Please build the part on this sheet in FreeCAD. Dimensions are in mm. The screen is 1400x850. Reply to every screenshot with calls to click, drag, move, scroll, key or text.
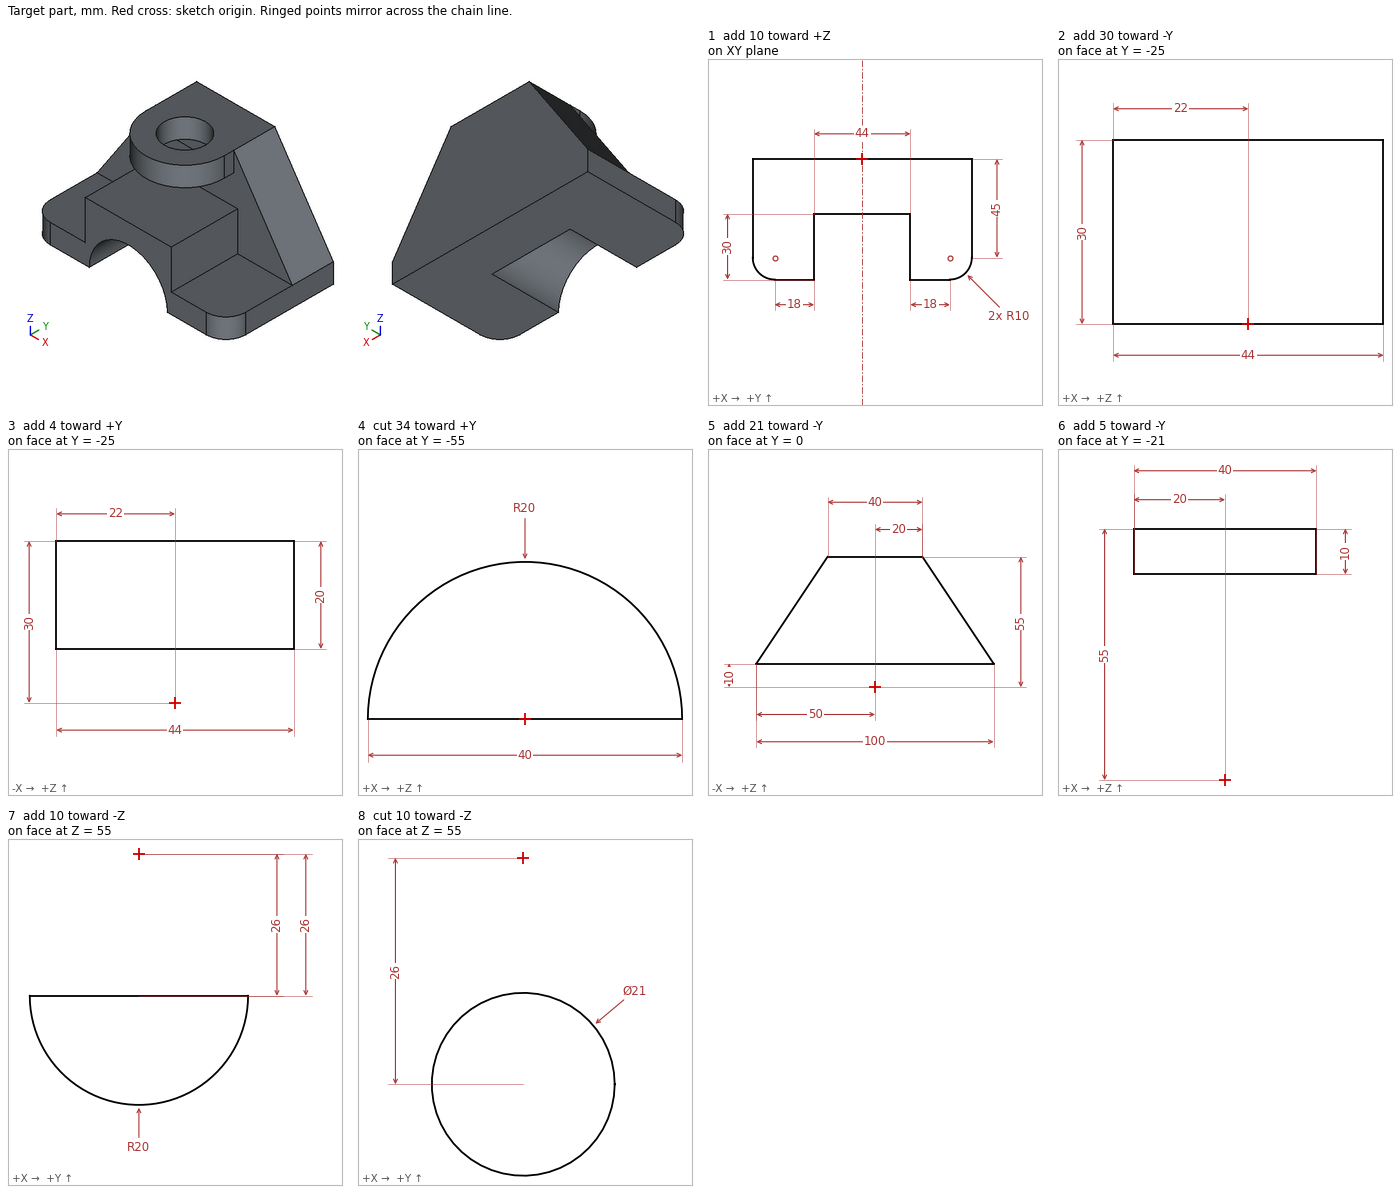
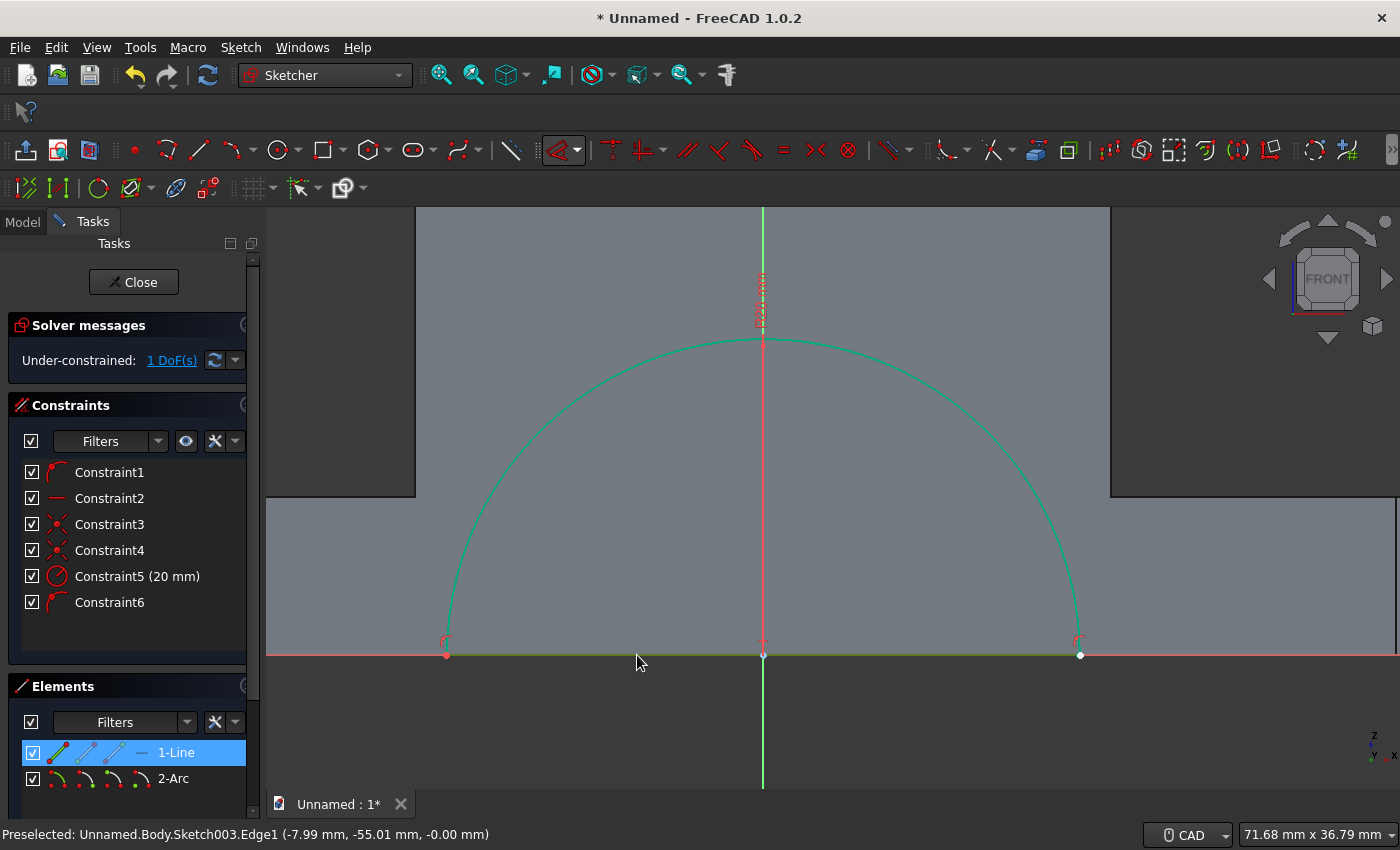
click(580, 150)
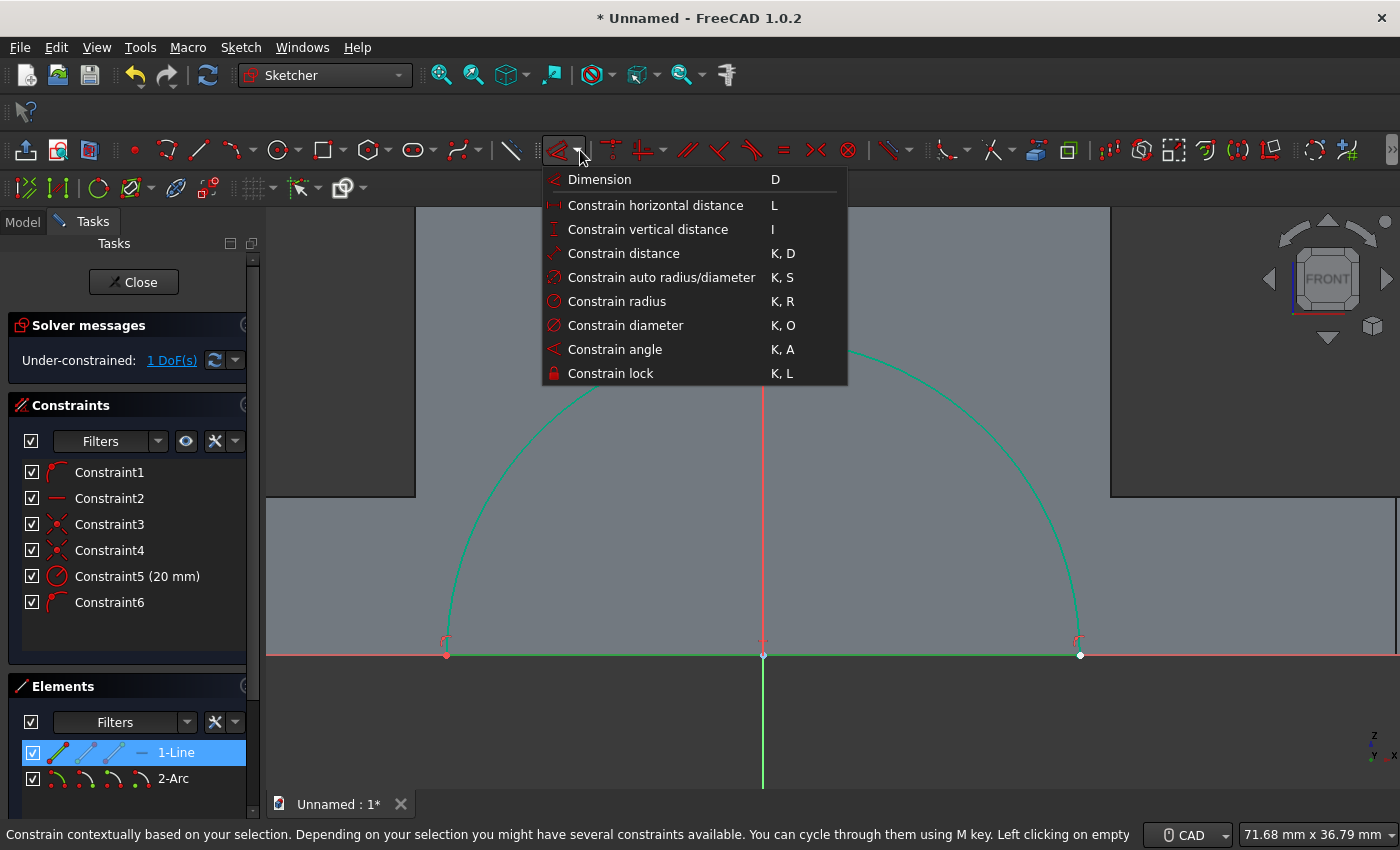
click(695, 205)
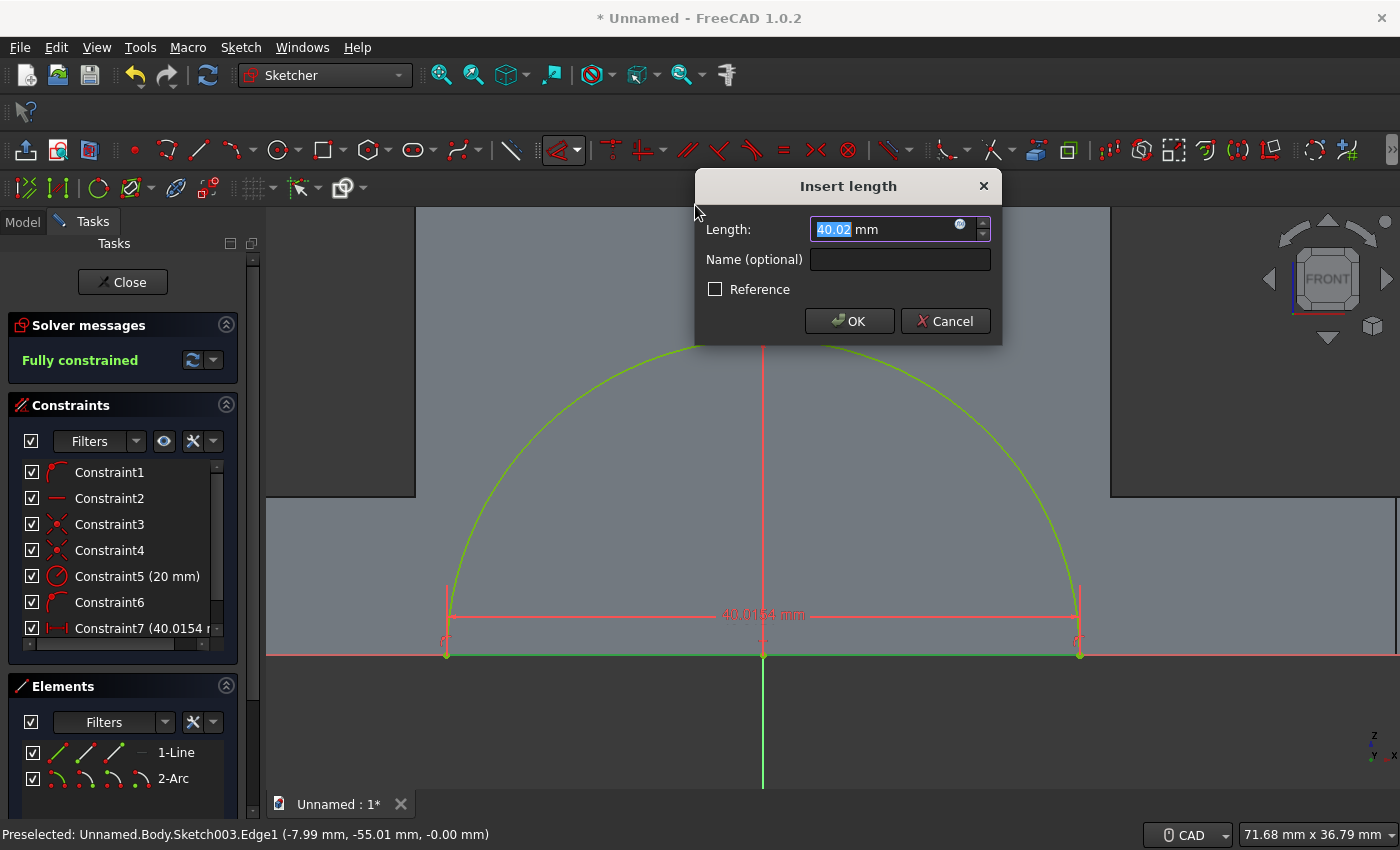
text(40)
key(Return)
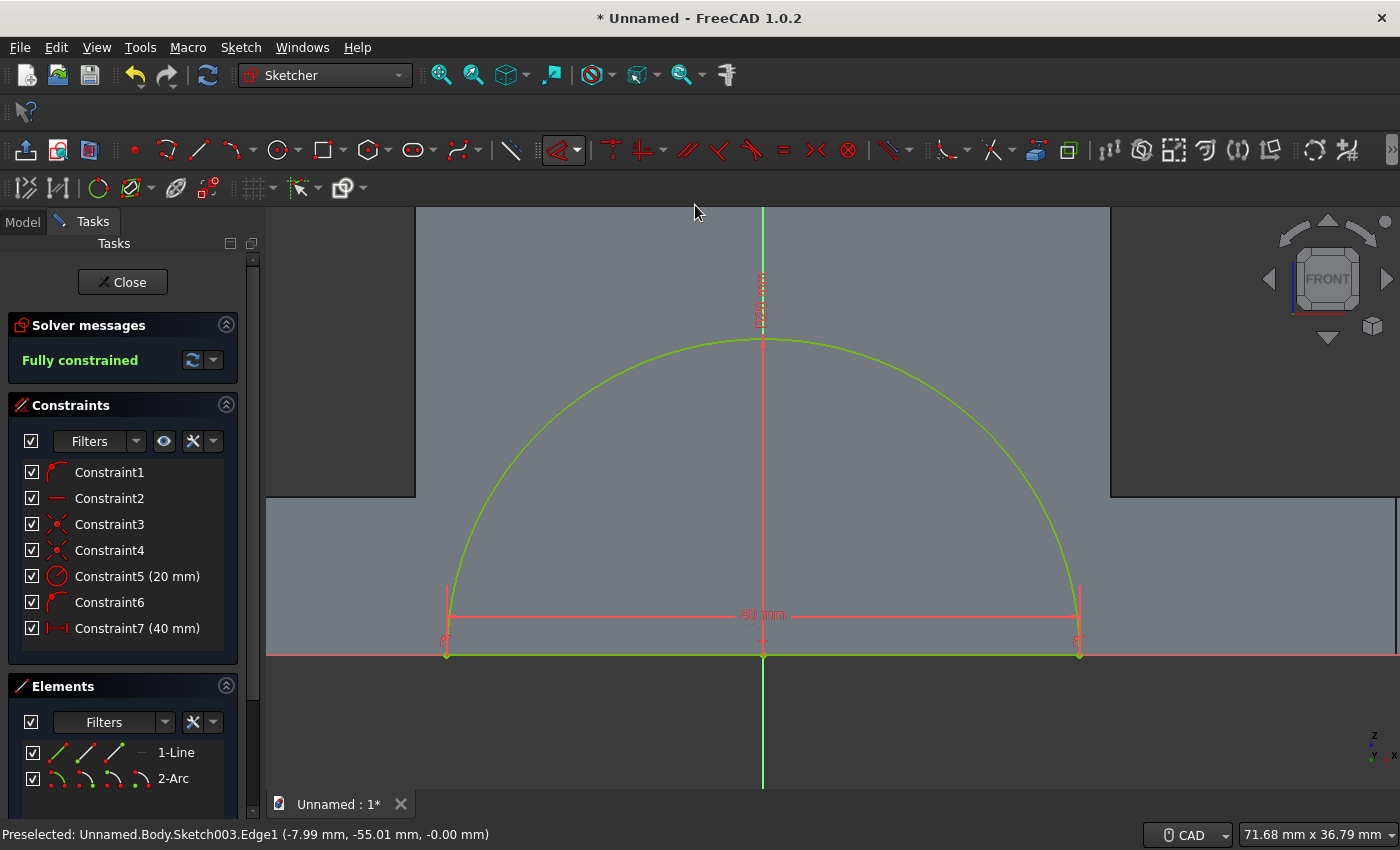
click(123, 282)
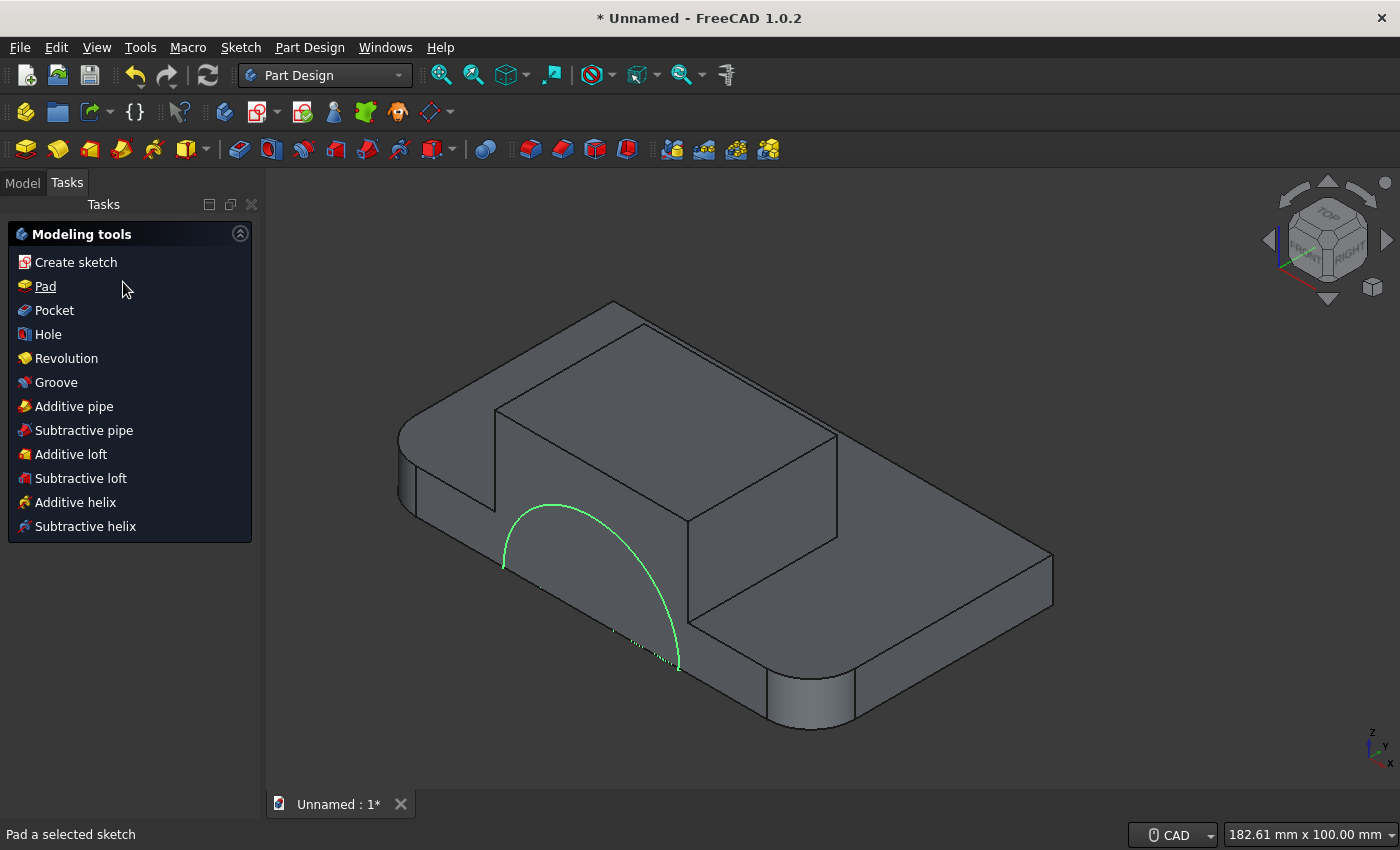
click(240, 150)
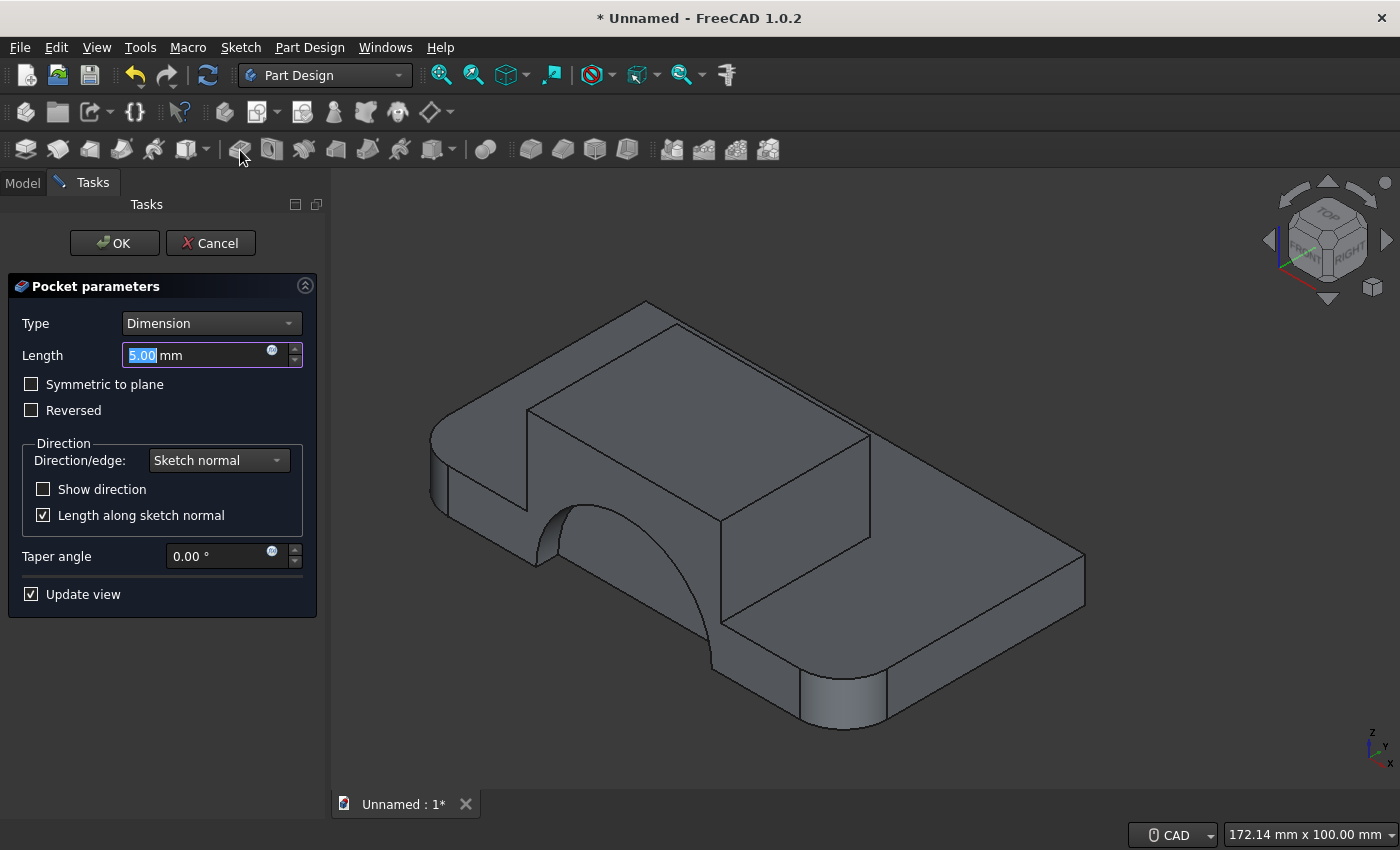
text(34)
key(Tab)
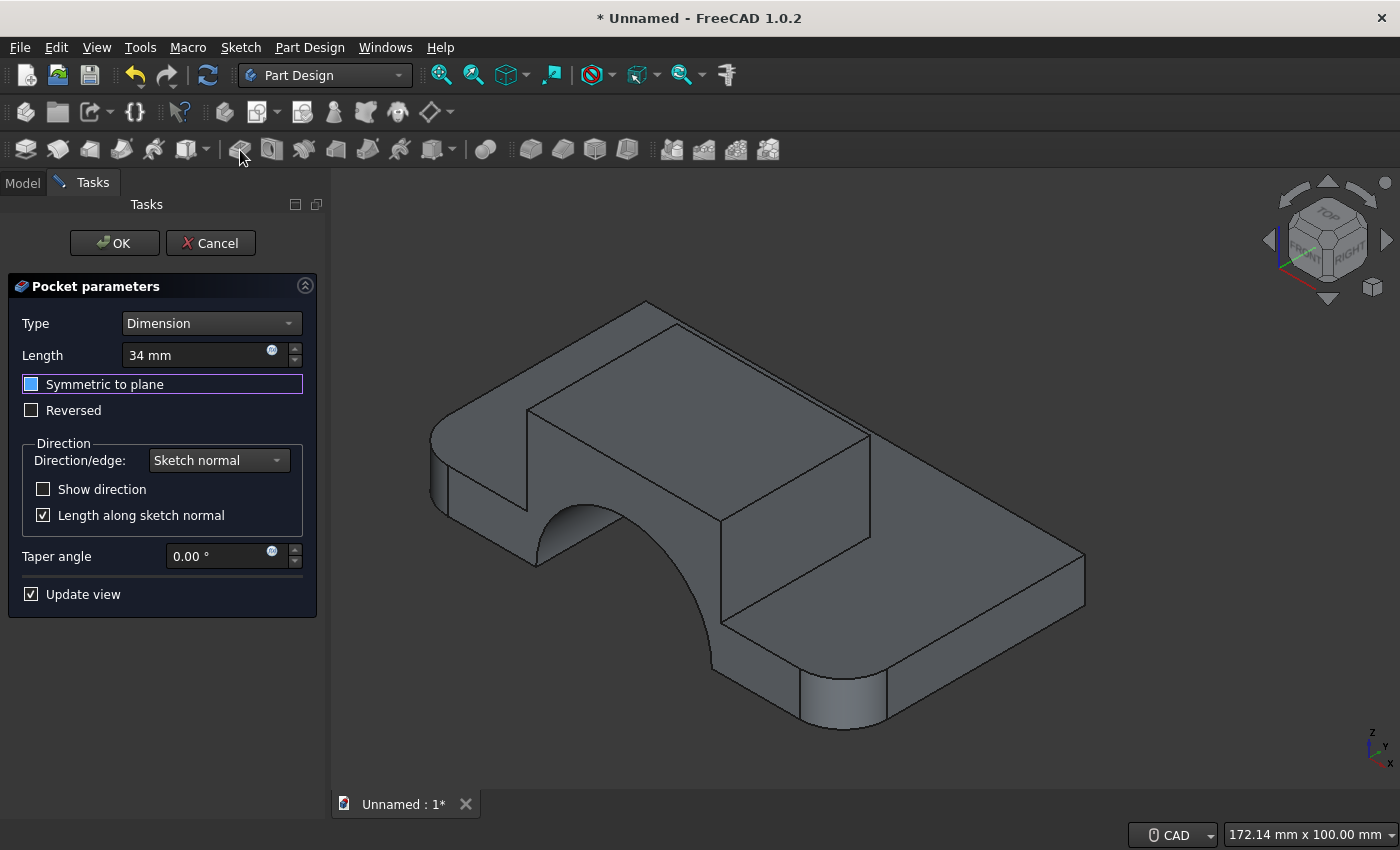
click(115, 243)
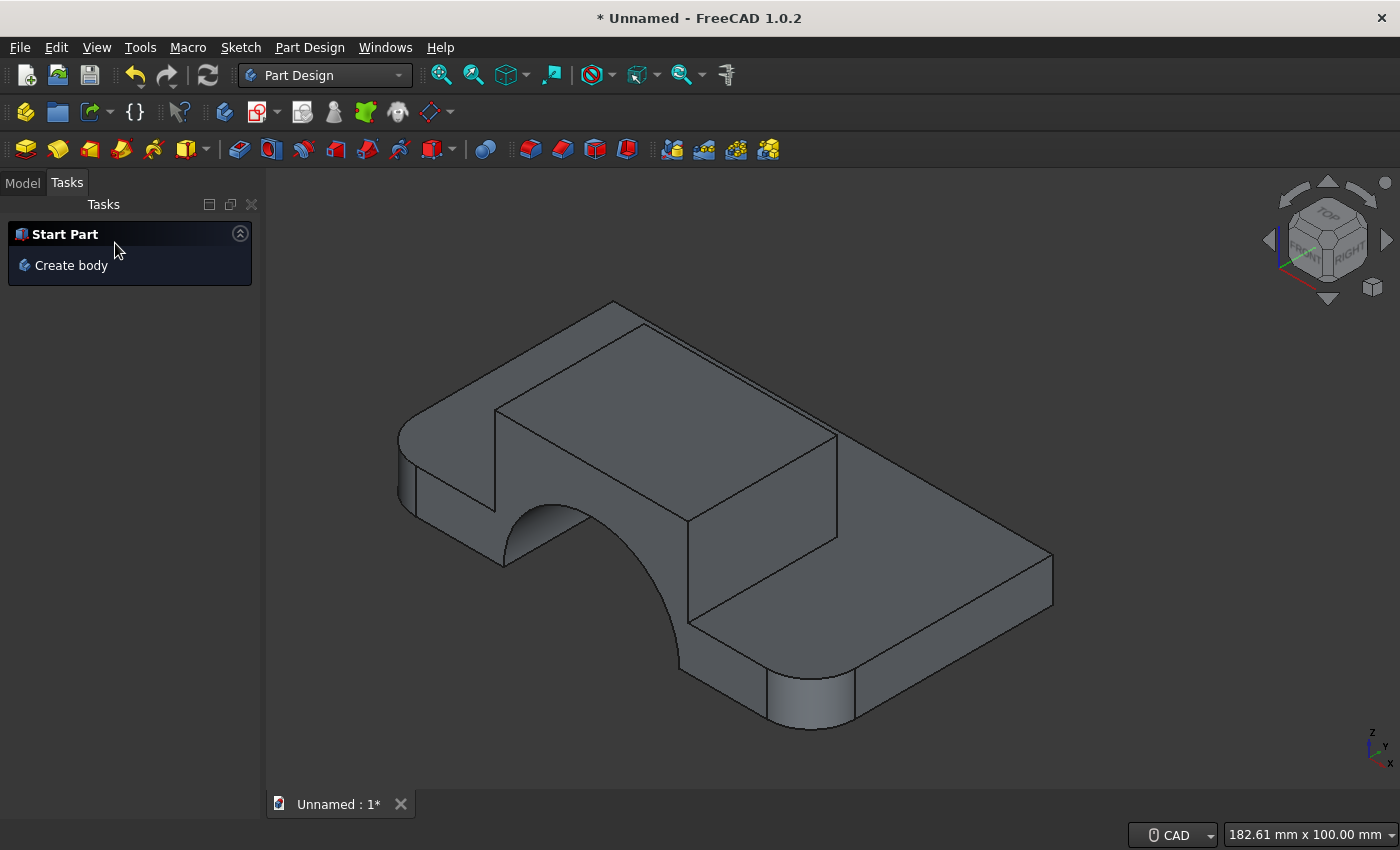
key(4)